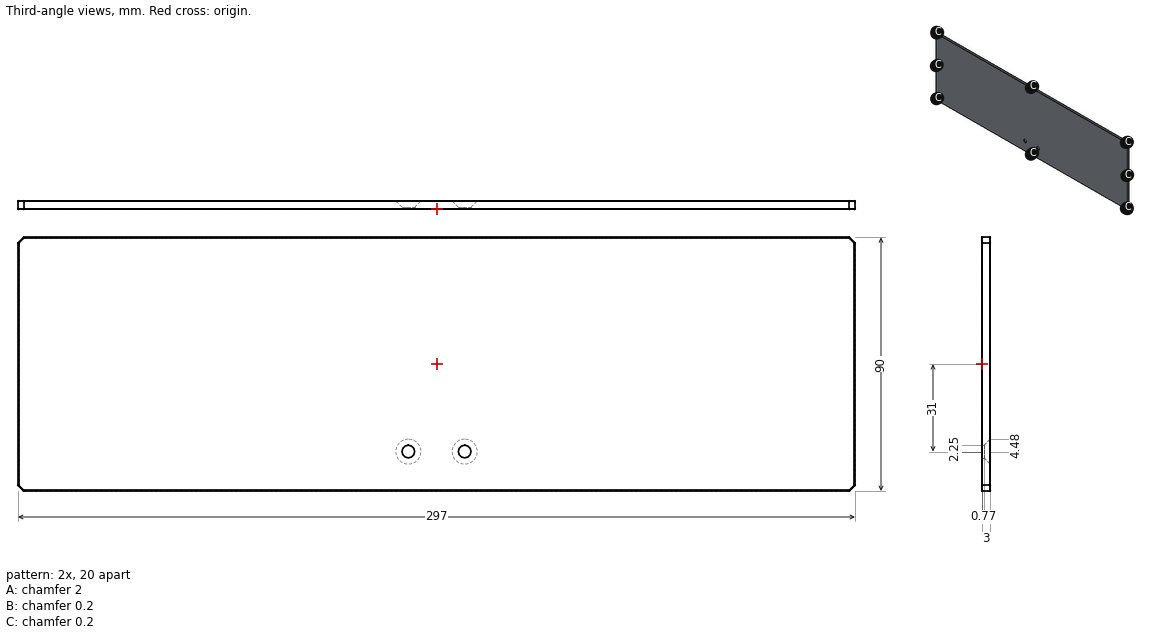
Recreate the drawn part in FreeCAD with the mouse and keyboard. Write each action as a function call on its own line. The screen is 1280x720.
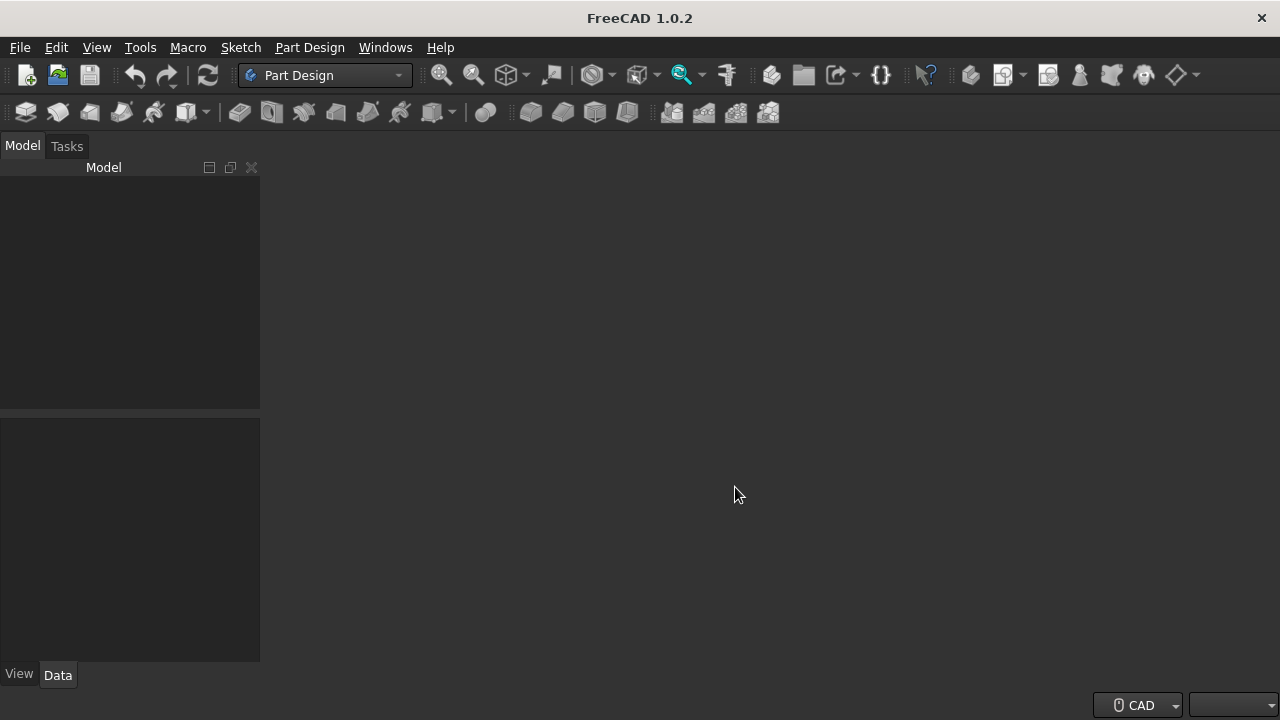
click(26, 76)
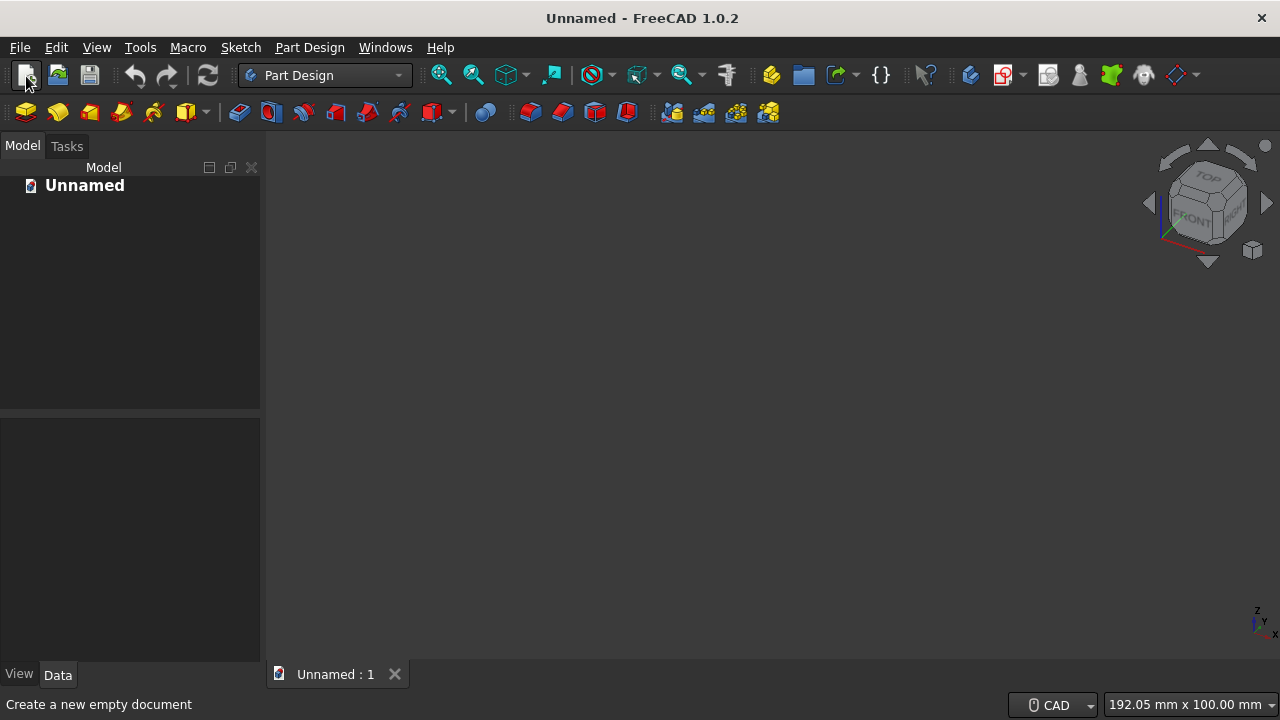
click(1004, 76)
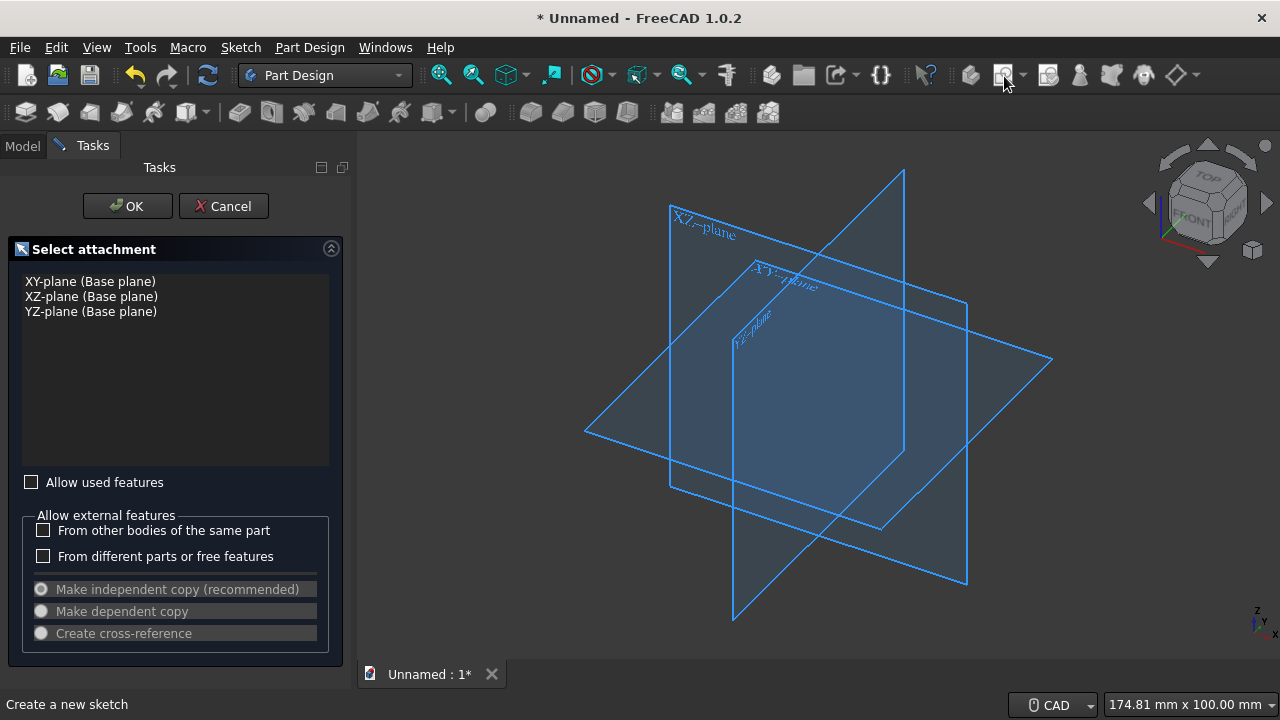
click(82, 296)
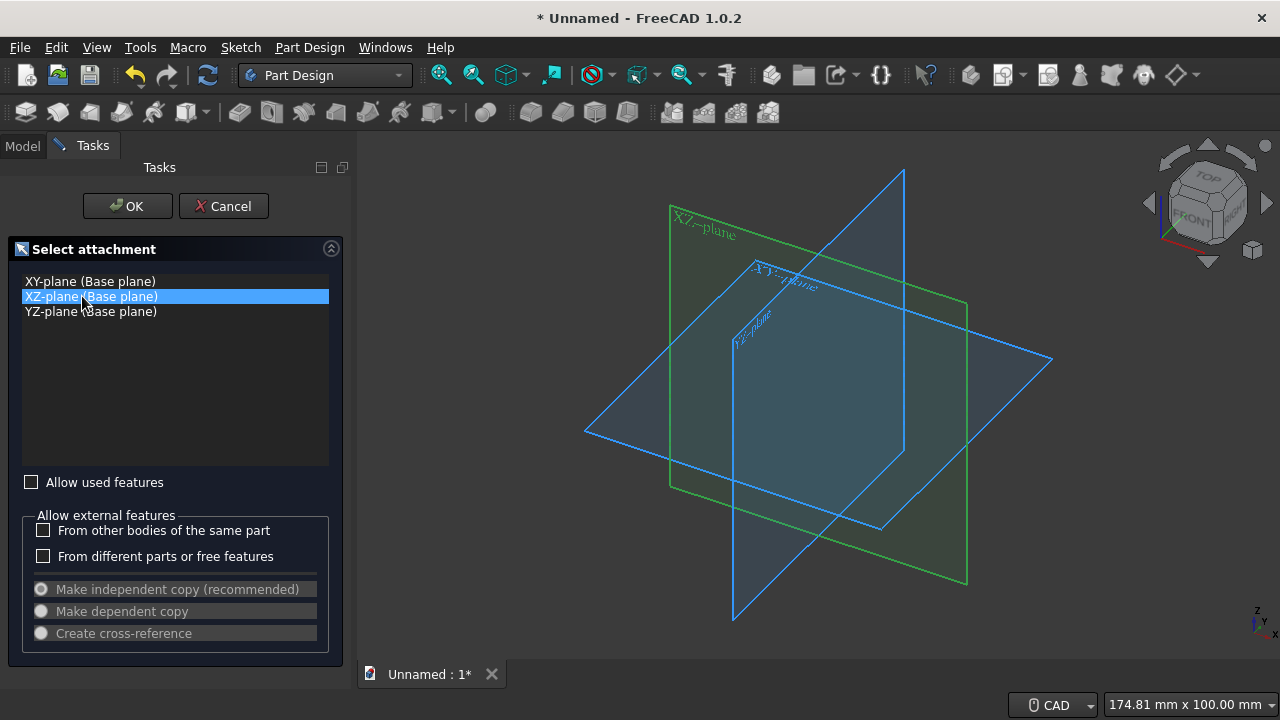
click(128, 206)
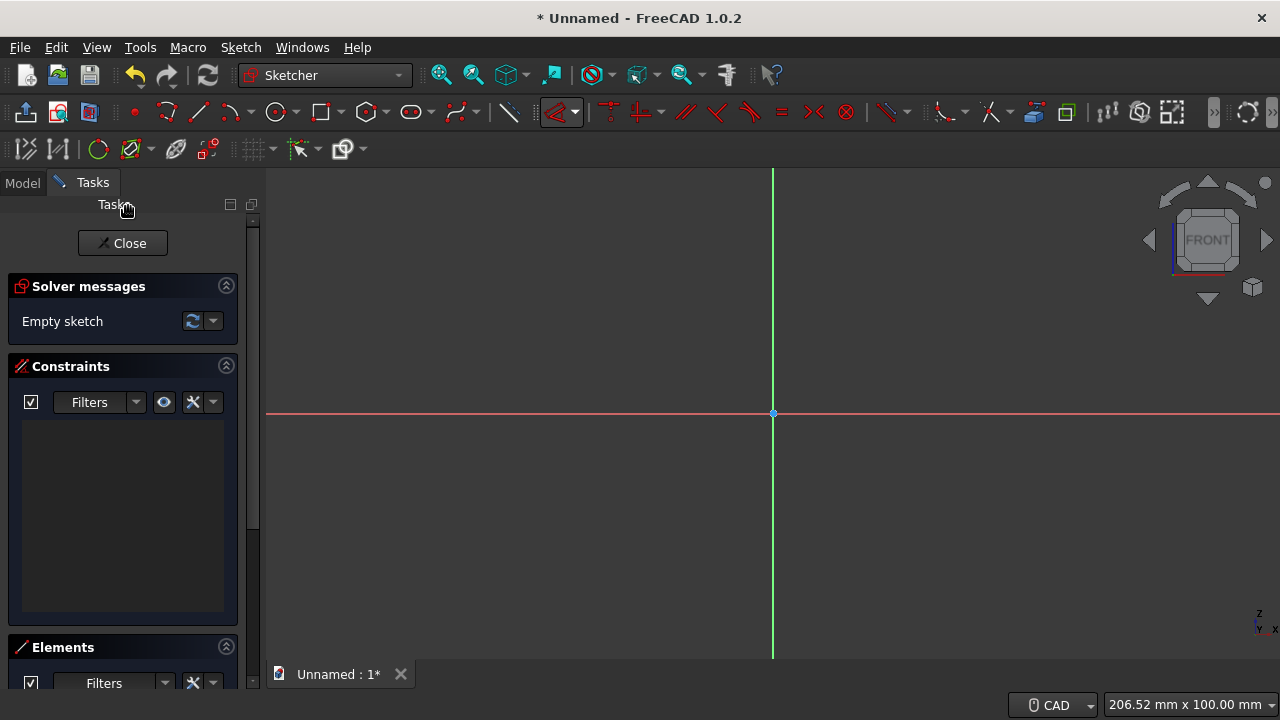
scroll(665, 414, down, 5)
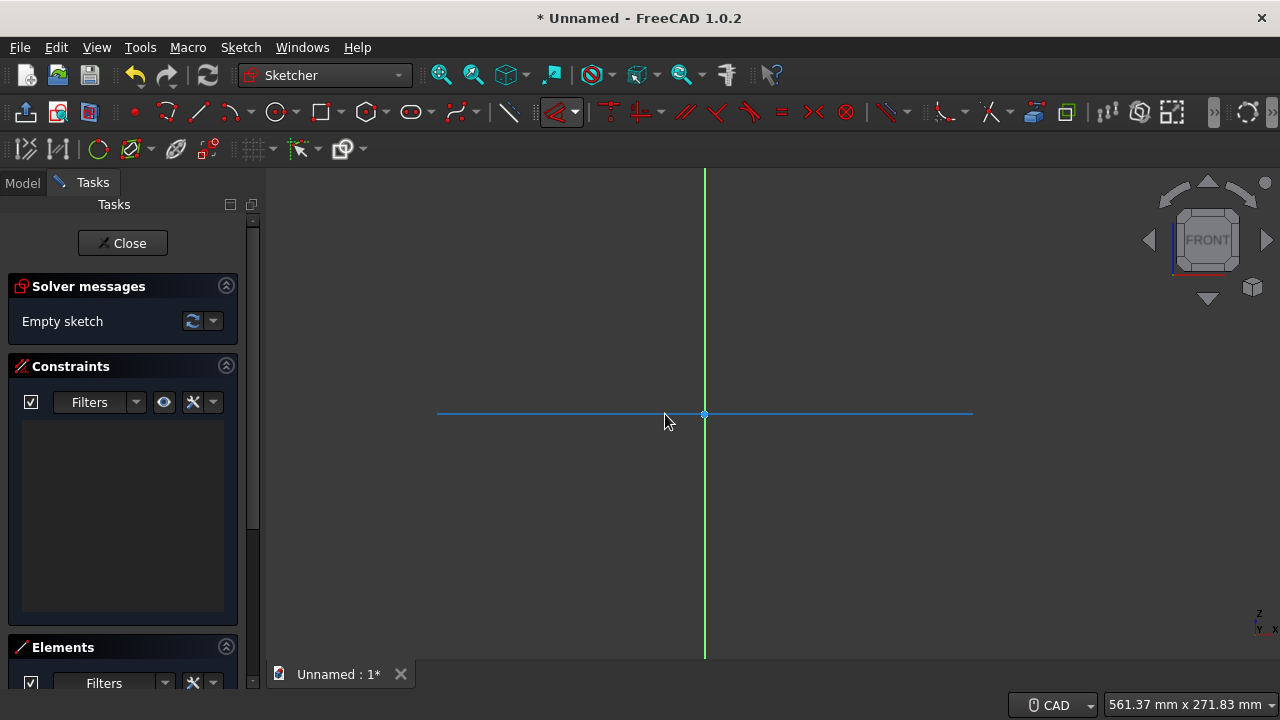
key(g)
key(v)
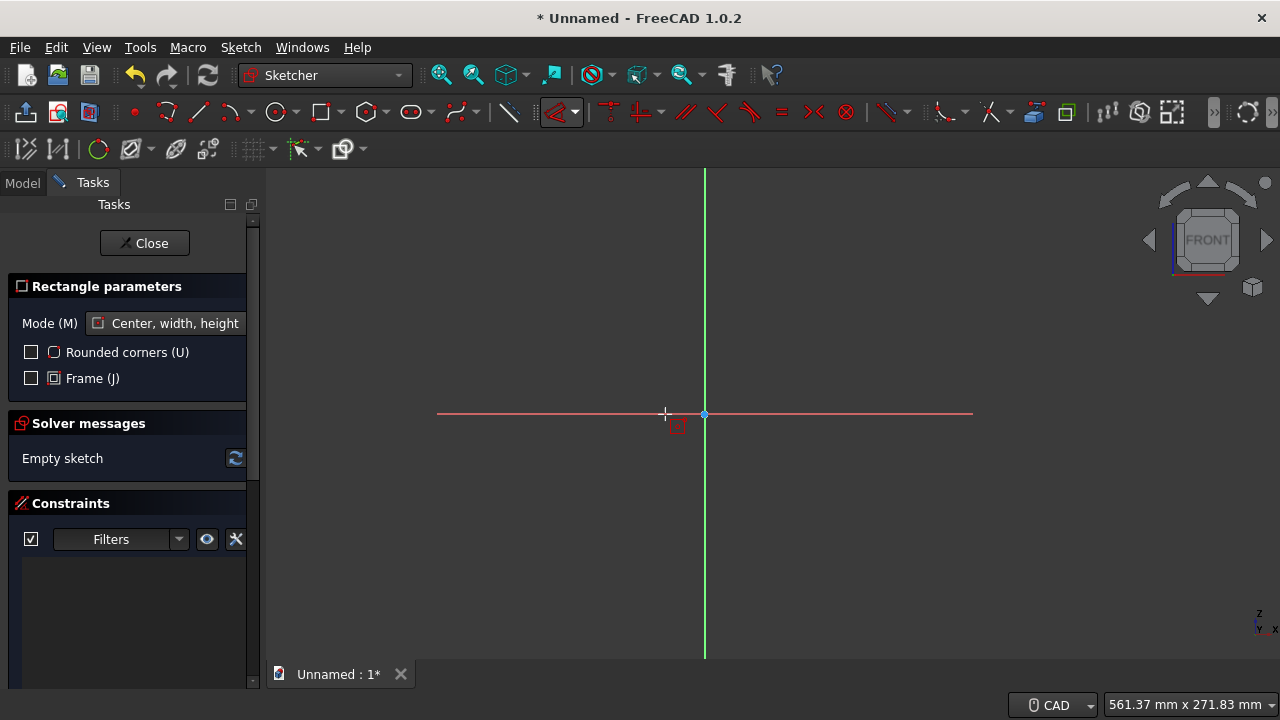
click(705, 414)
click(973, 333)
key(Escape)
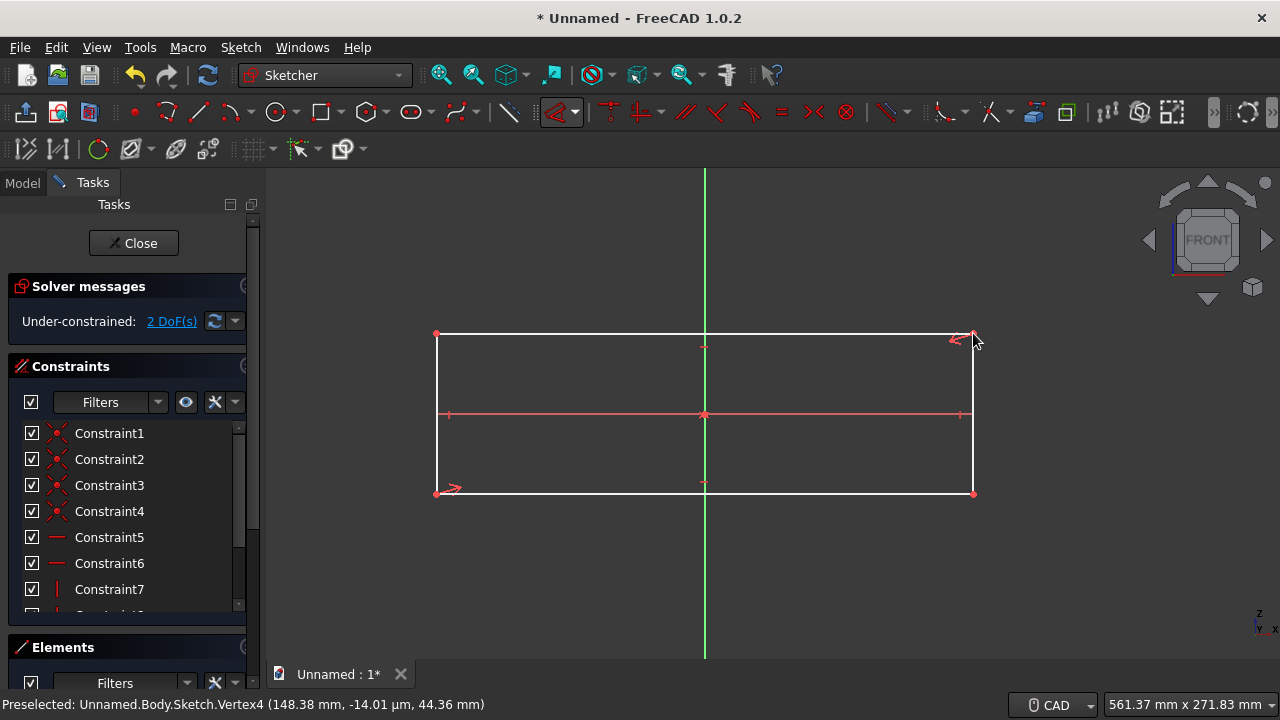
click(973, 446)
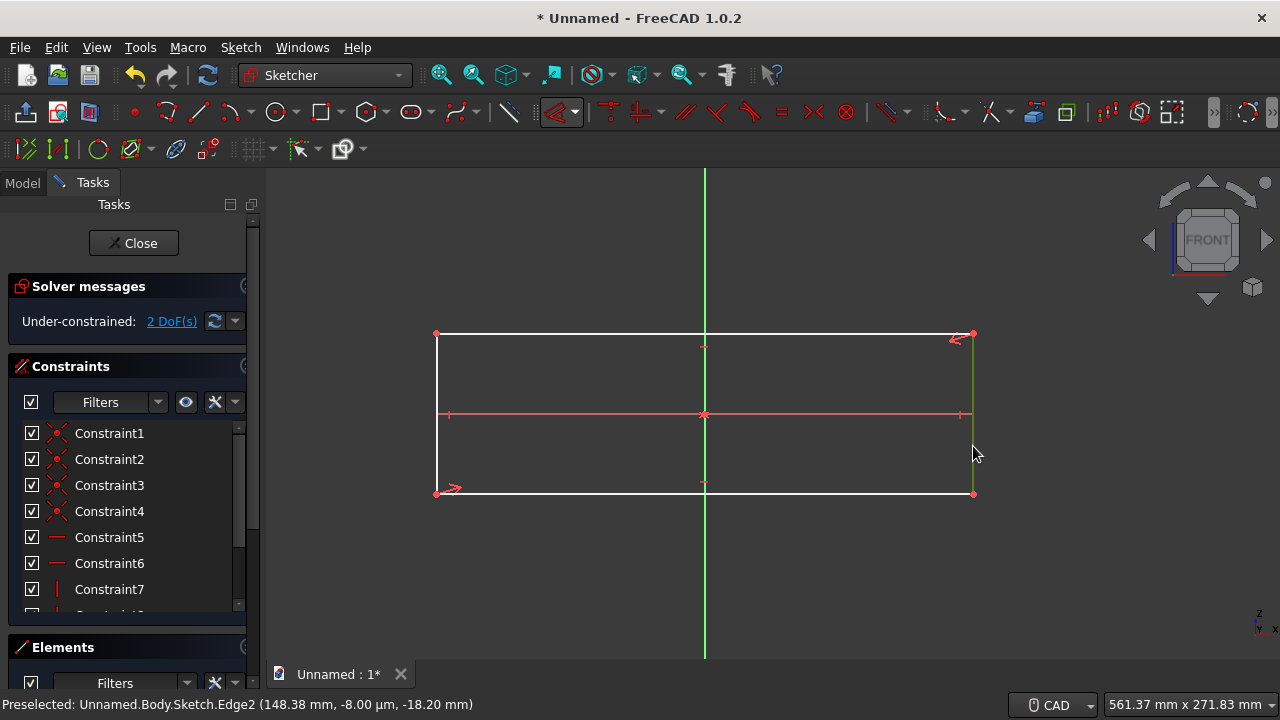
key(i)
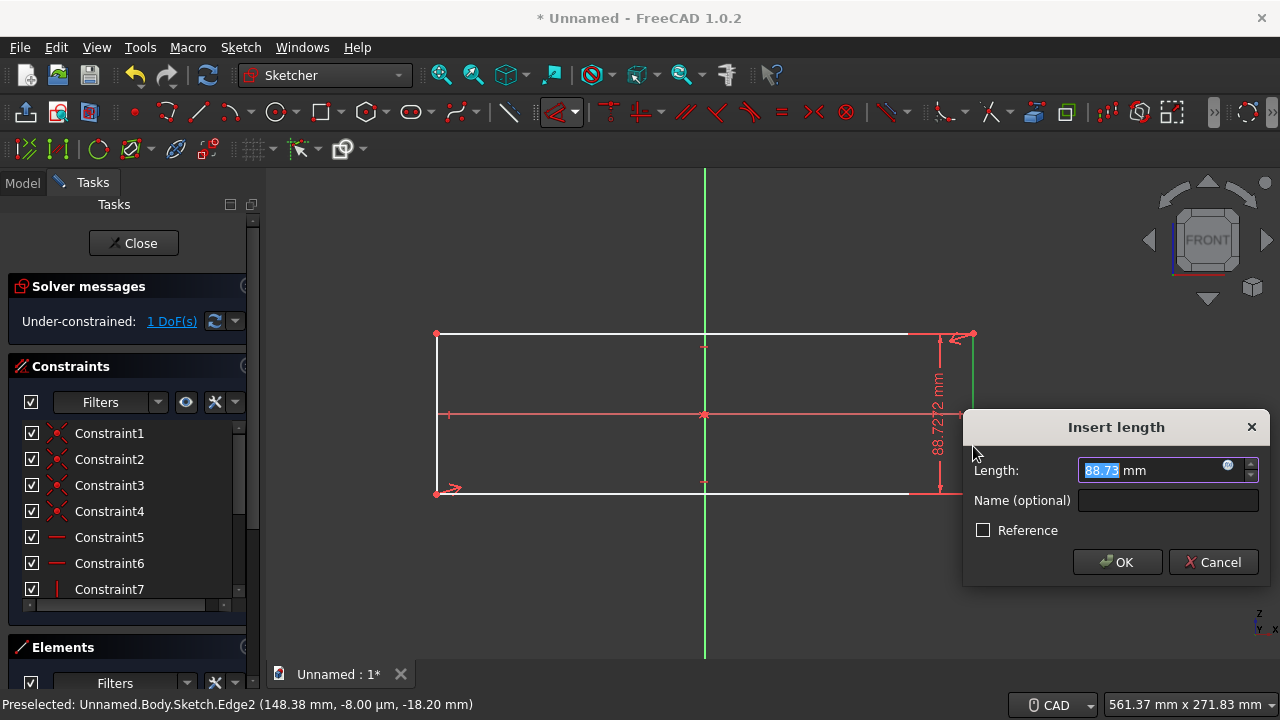
text(90)
key(Return)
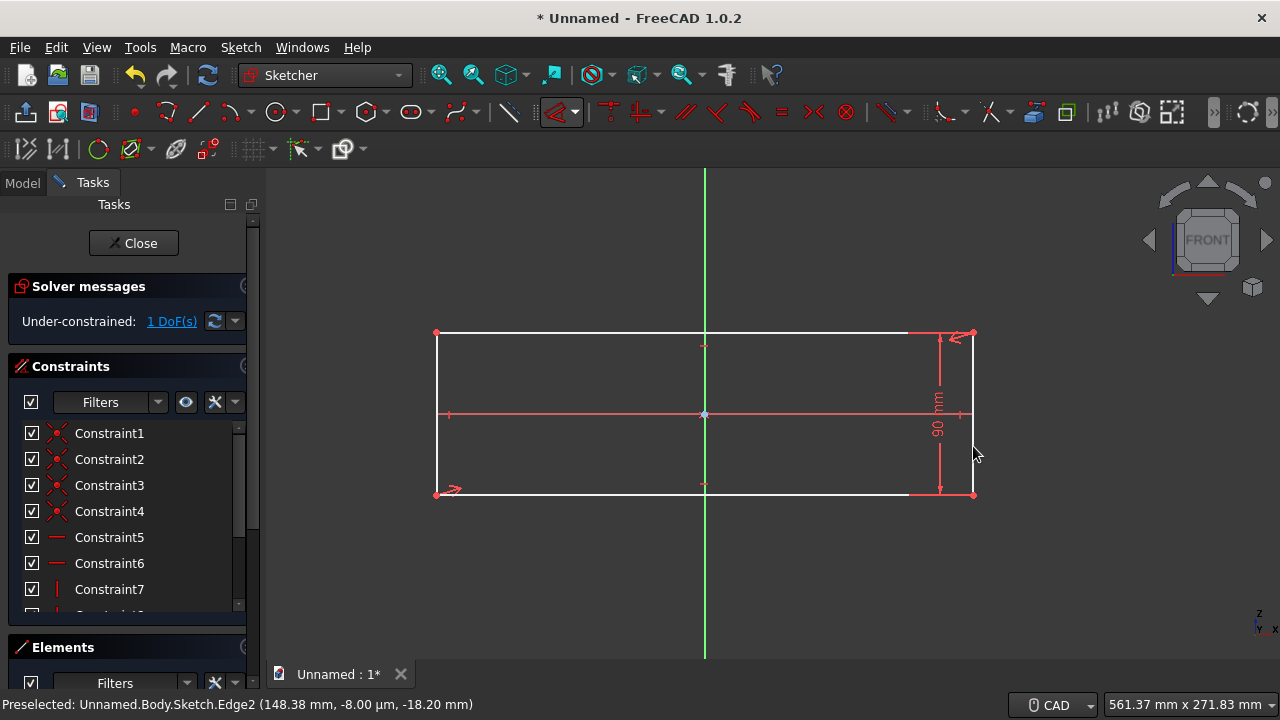
click(598, 495)